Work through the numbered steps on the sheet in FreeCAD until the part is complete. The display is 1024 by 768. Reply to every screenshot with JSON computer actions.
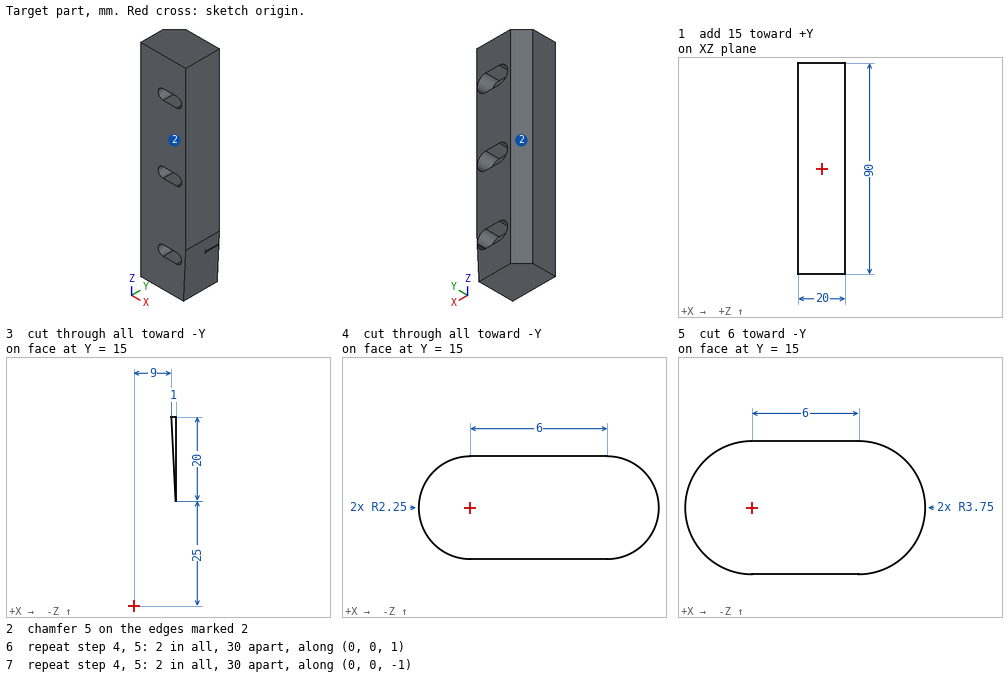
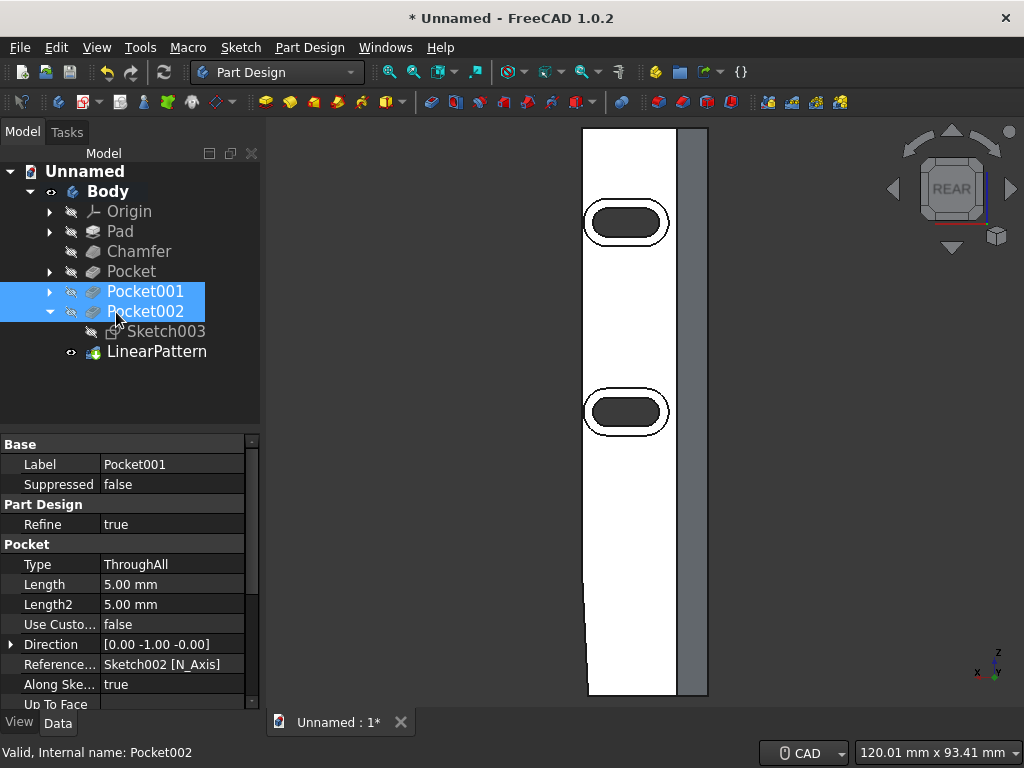
{"action": "left_click", "coordinate": [792, 102]}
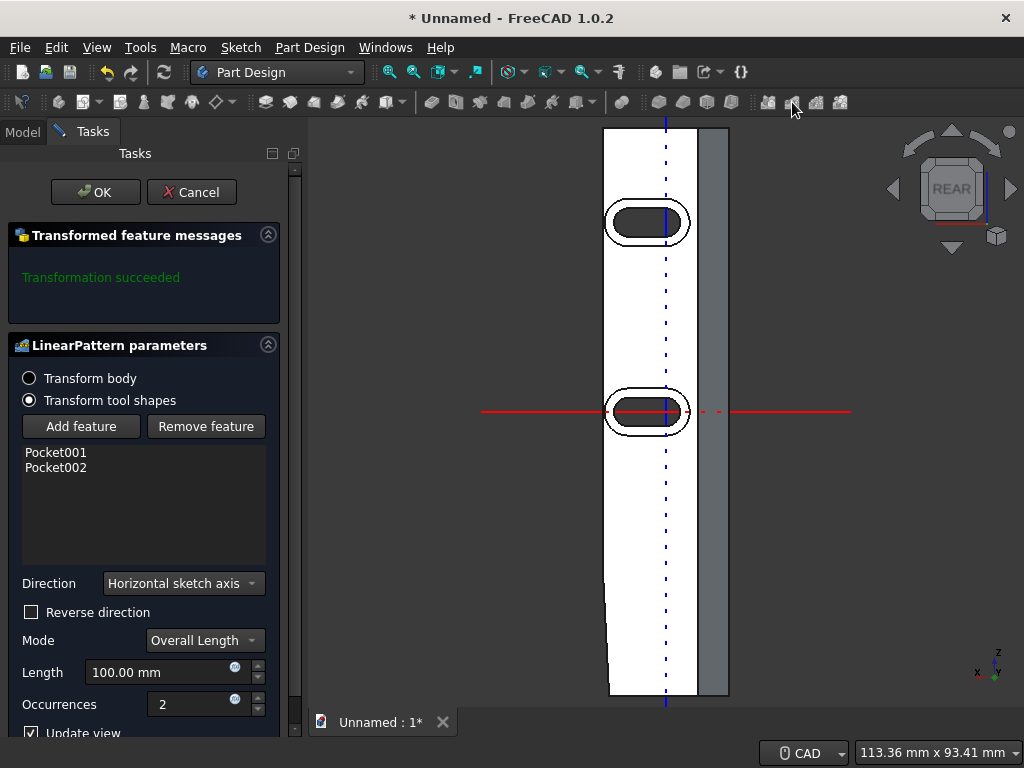
{"action": "left_click", "coordinate": [184, 584]}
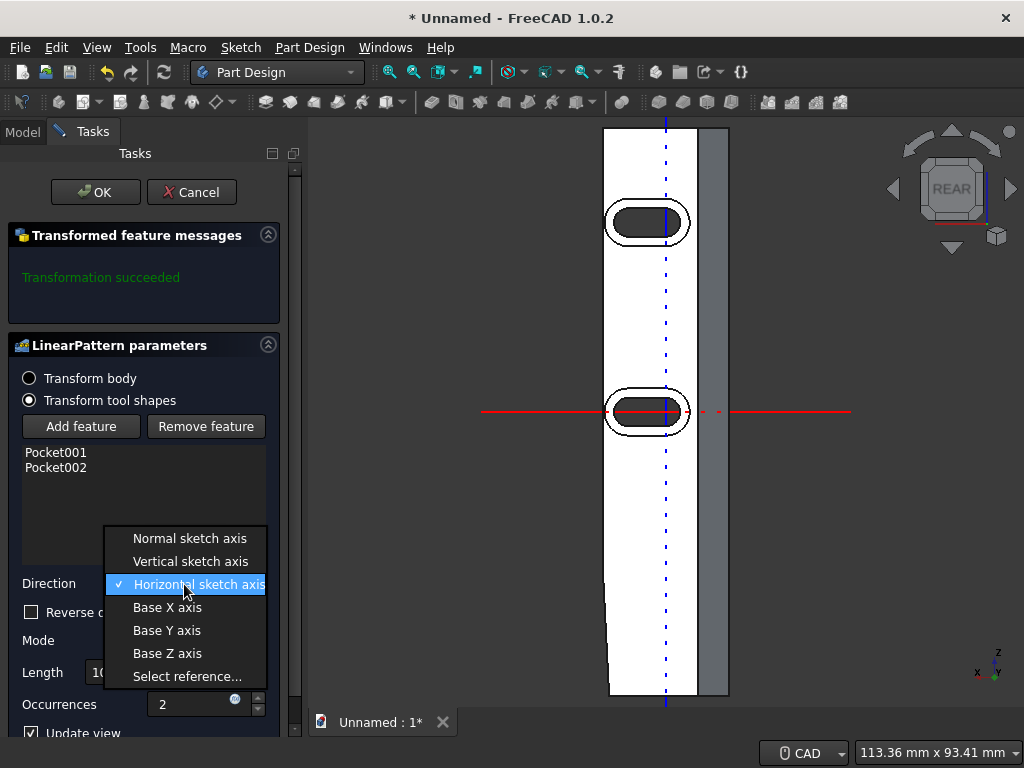
{"action": "left_click", "coordinate": [184, 654]}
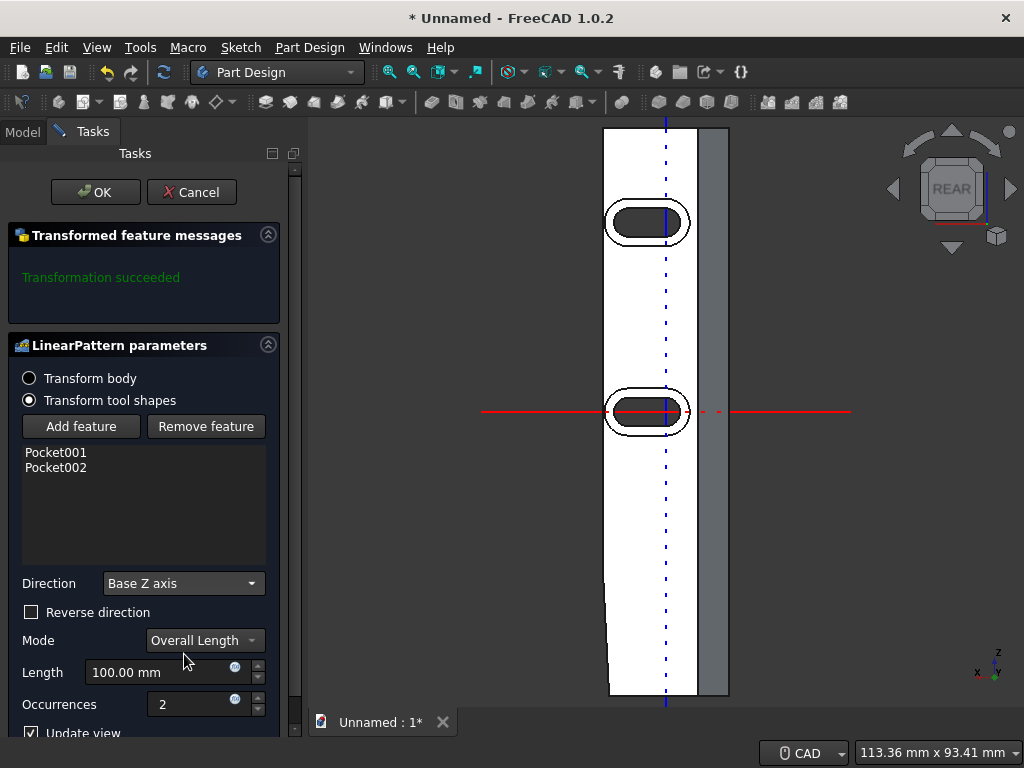
{"action": "left_click", "coordinate": [206, 640]}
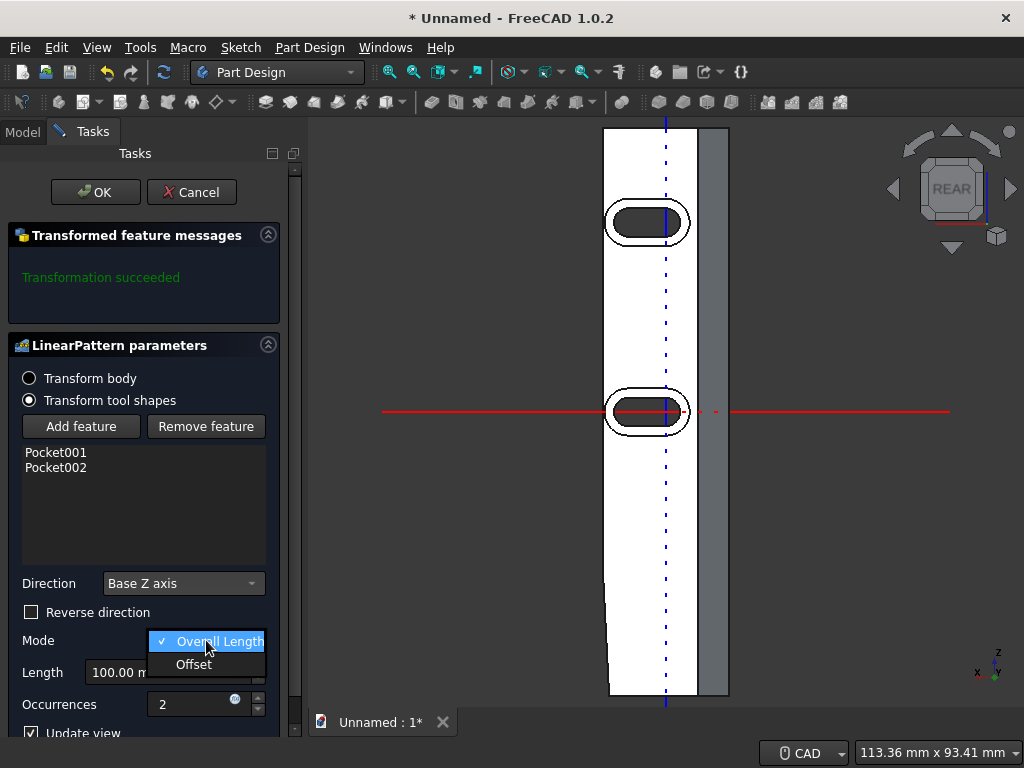
{"action": "left_click", "coordinate": [206, 664]}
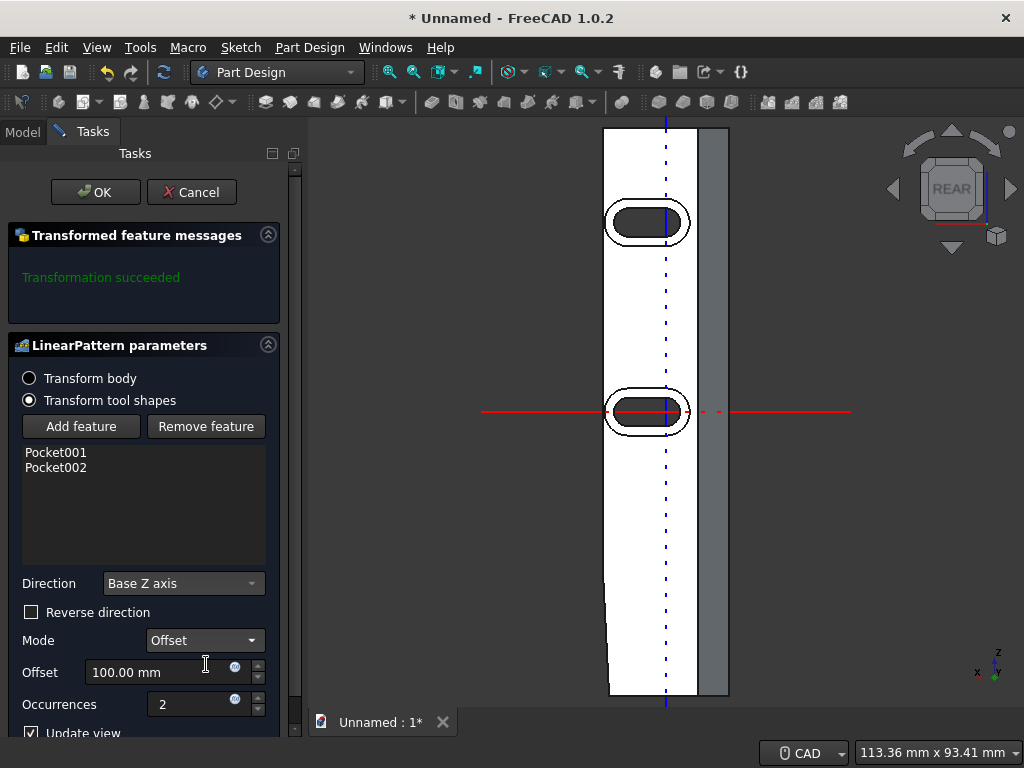
{"action": "triple_click", "coordinate": [168, 672]}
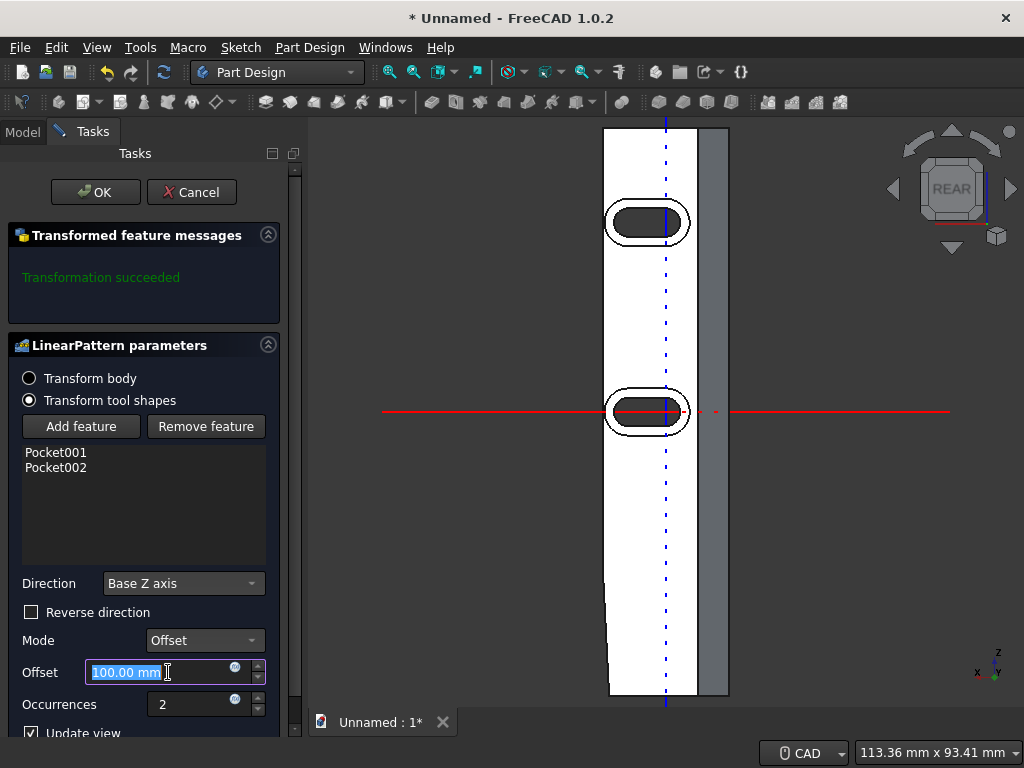
{"action": "type", "text": "30"}
{"action": "key", "text": "Tab"}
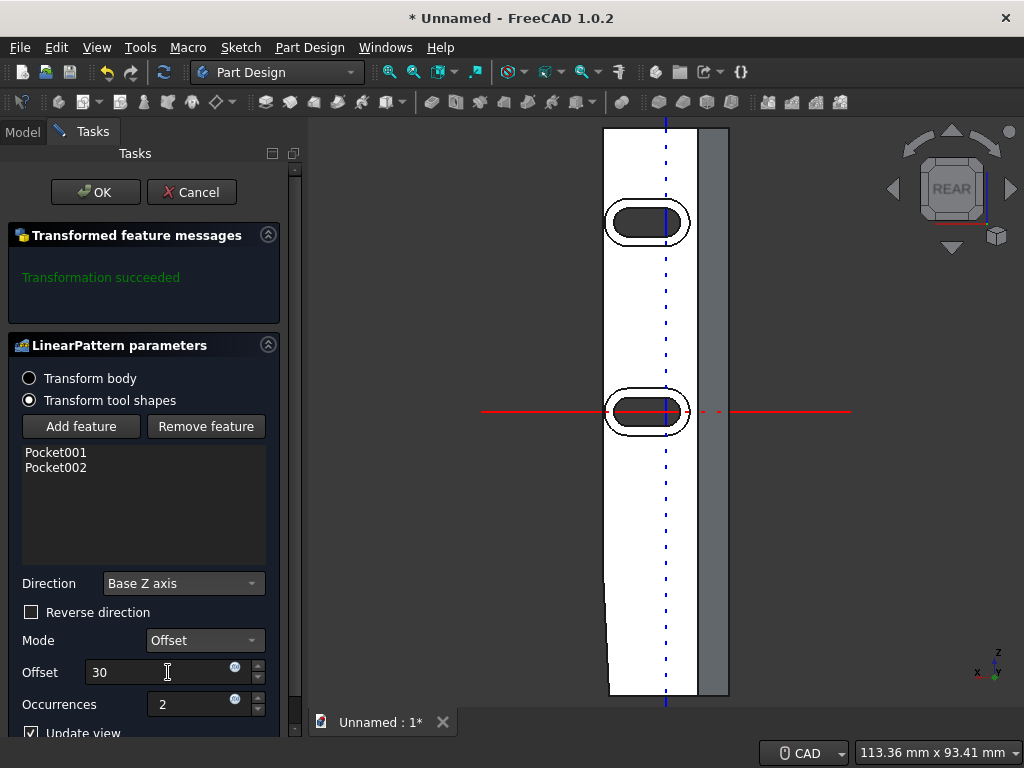
{"action": "triple_click", "coordinate": [198, 704]}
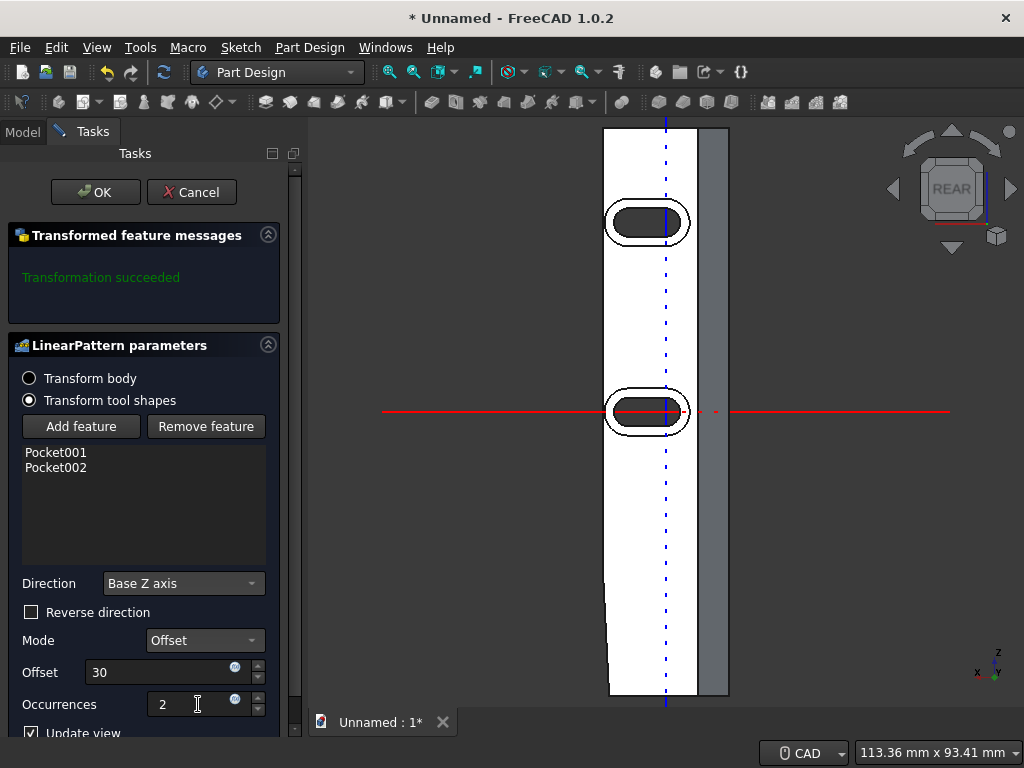
{"action": "type", "text": "2"}
{"action": "key", "text": "Tab"}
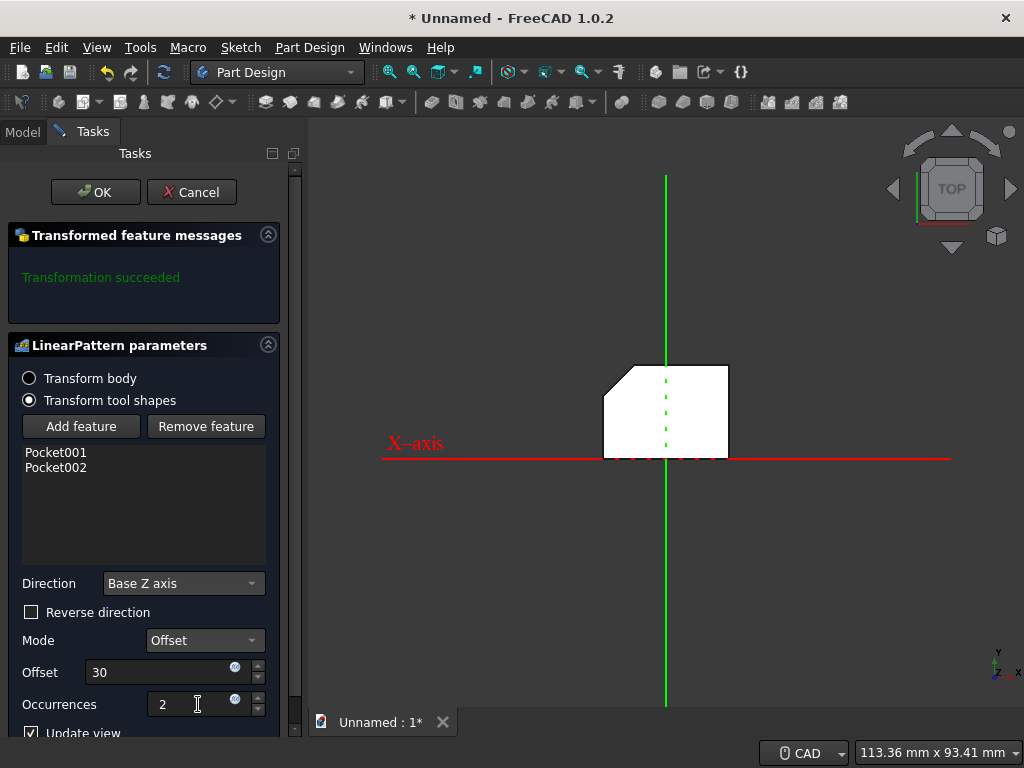
{"action": "left_click", "coordinate": [30, 612]}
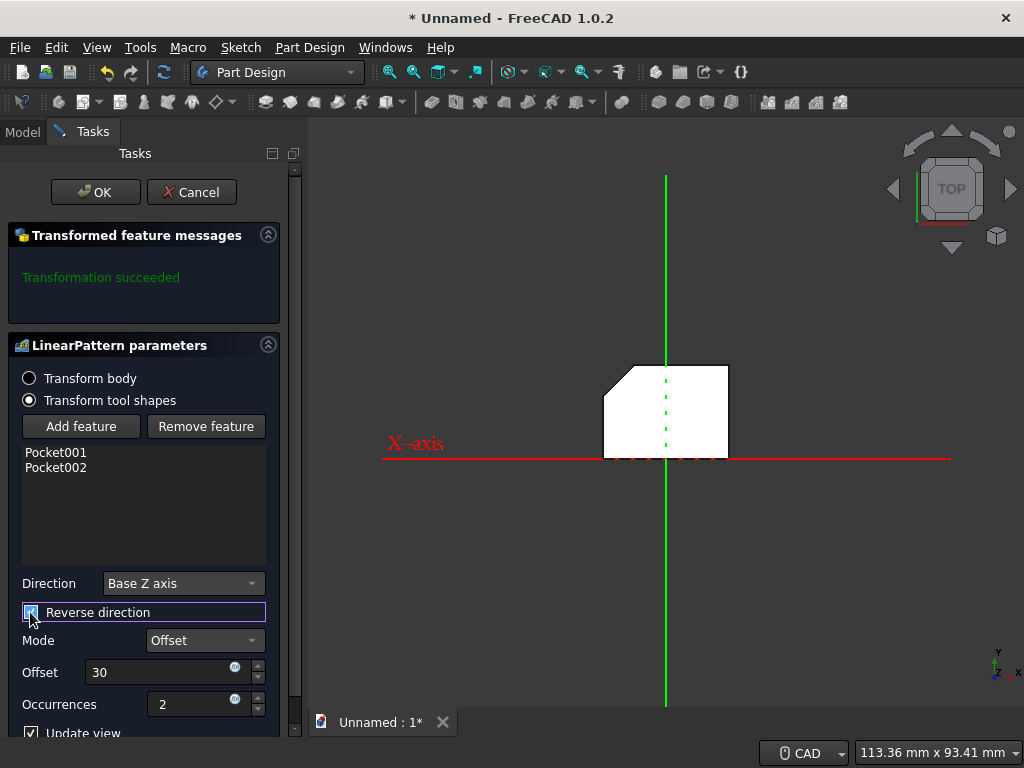
{"action": "left_click", "coordinate": [96, 192]}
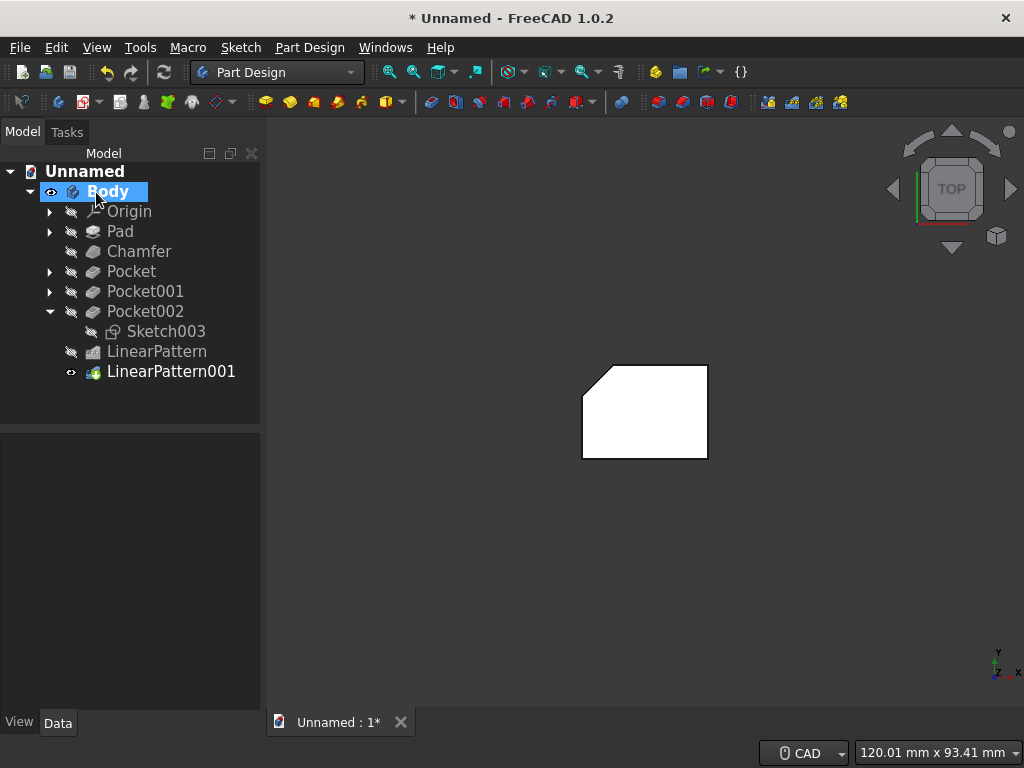
{"action": "key", "text": "0"}